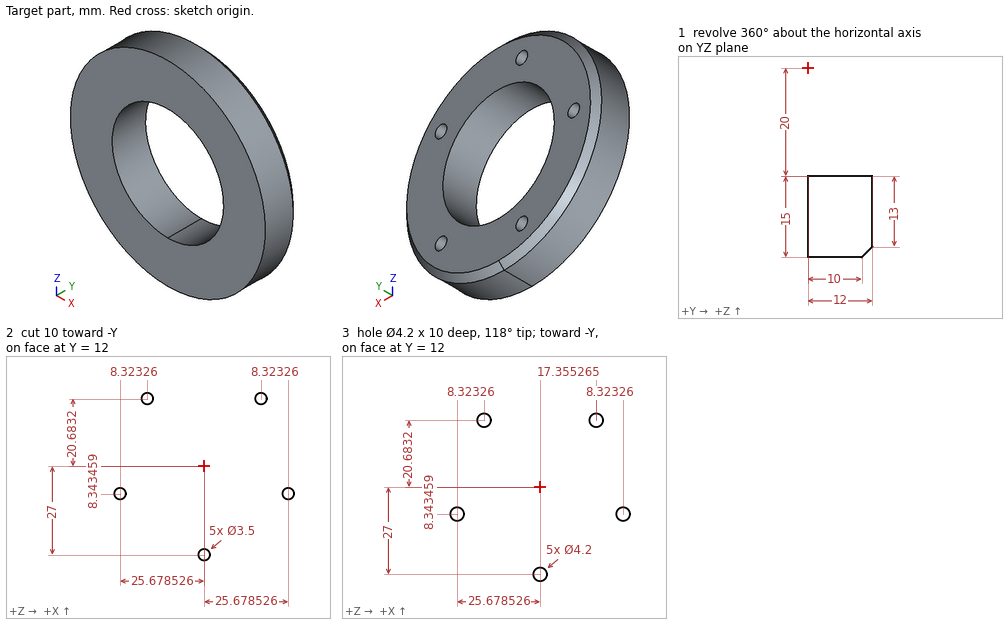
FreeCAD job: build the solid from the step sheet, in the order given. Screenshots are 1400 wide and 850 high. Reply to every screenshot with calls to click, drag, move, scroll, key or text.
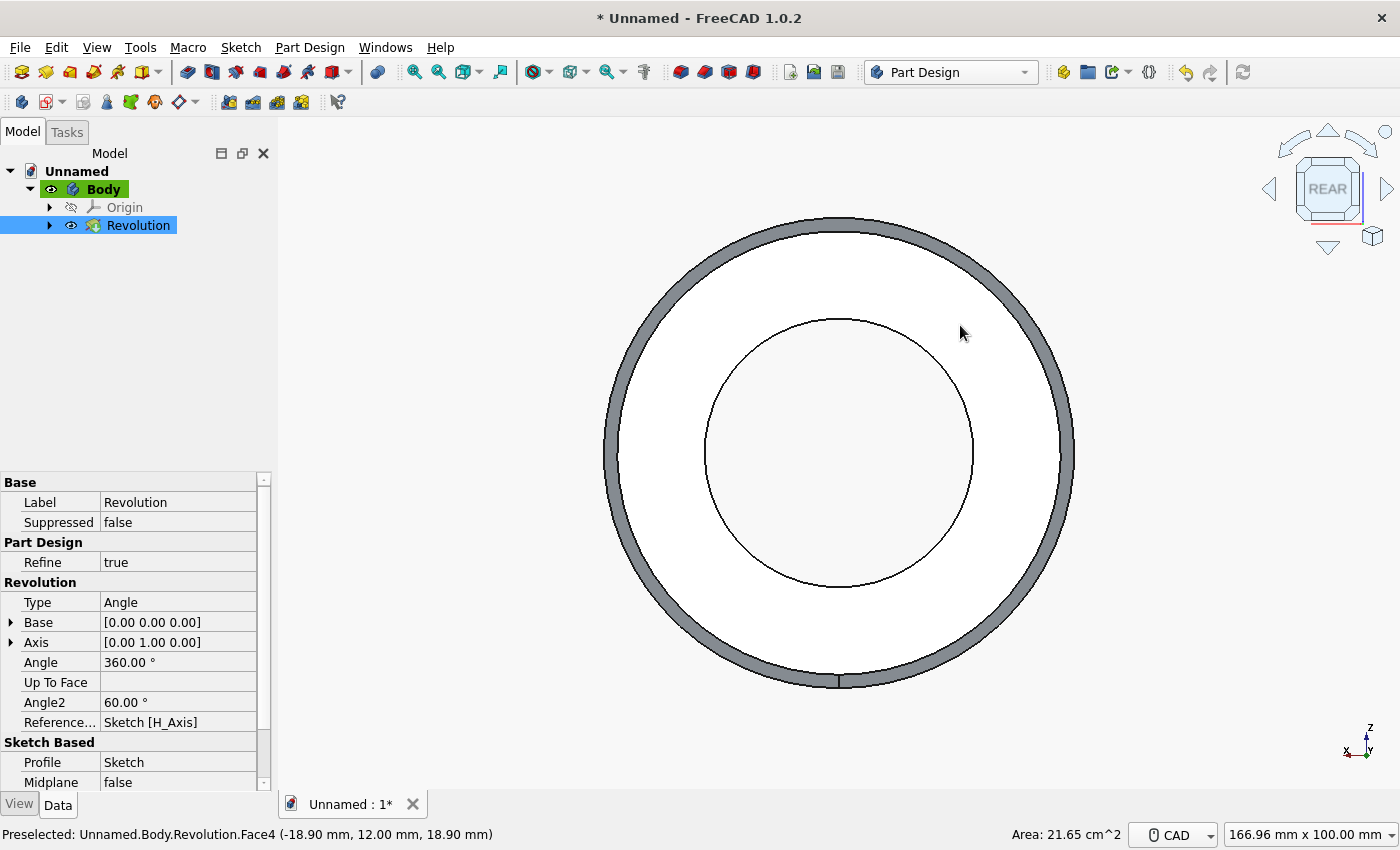
click(46, 102)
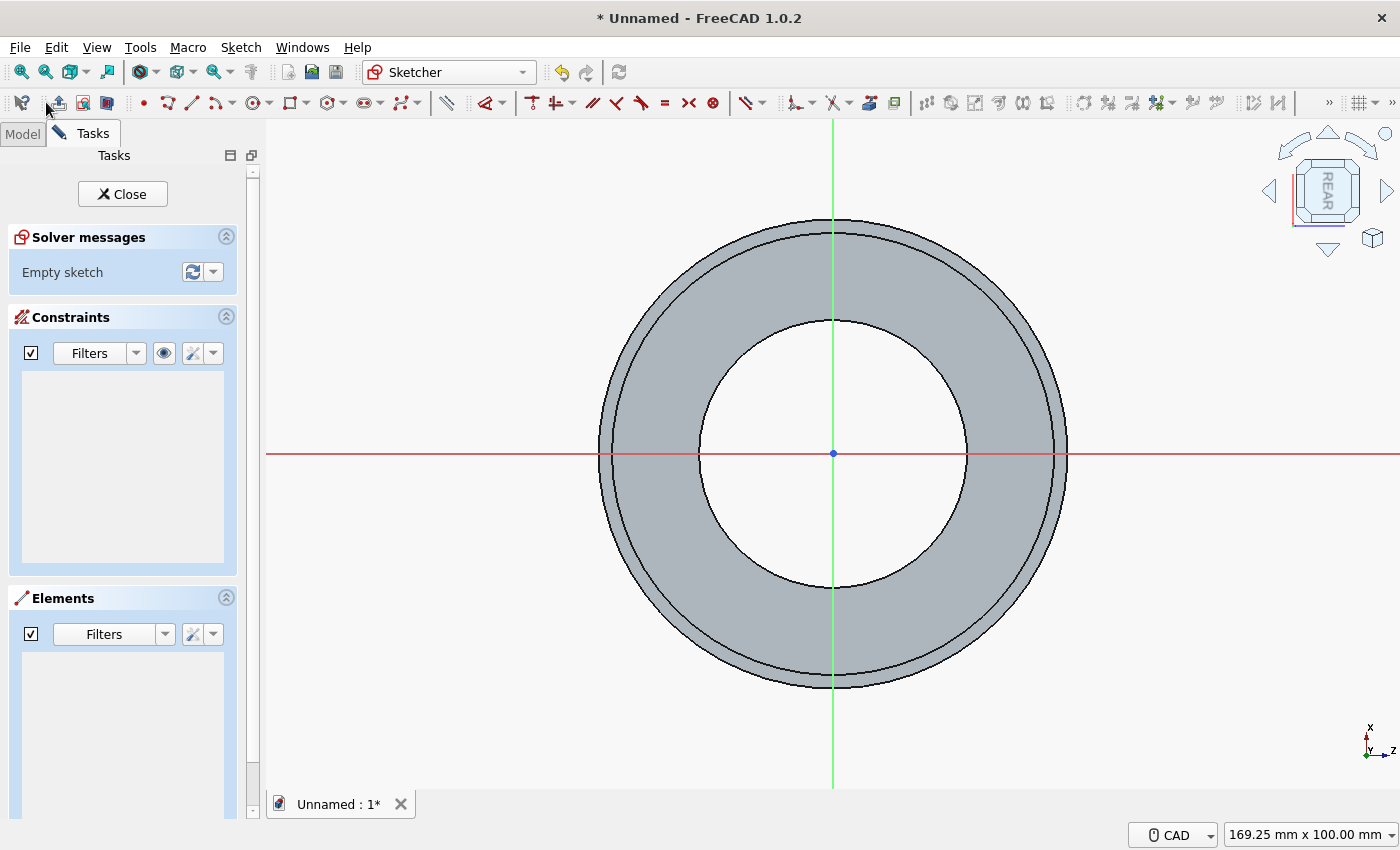
click(254, 104)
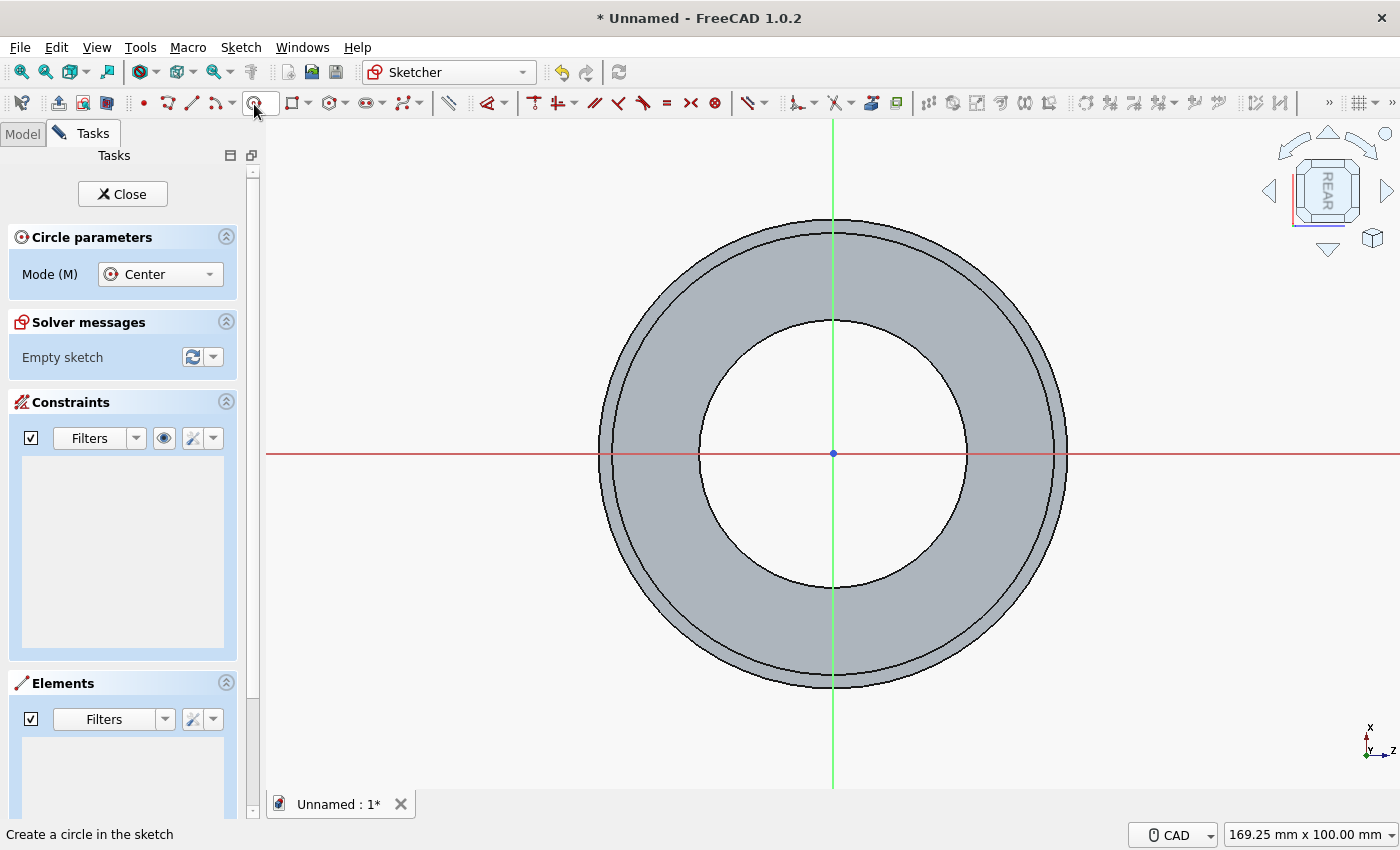
scroll(833, 635, up, 4)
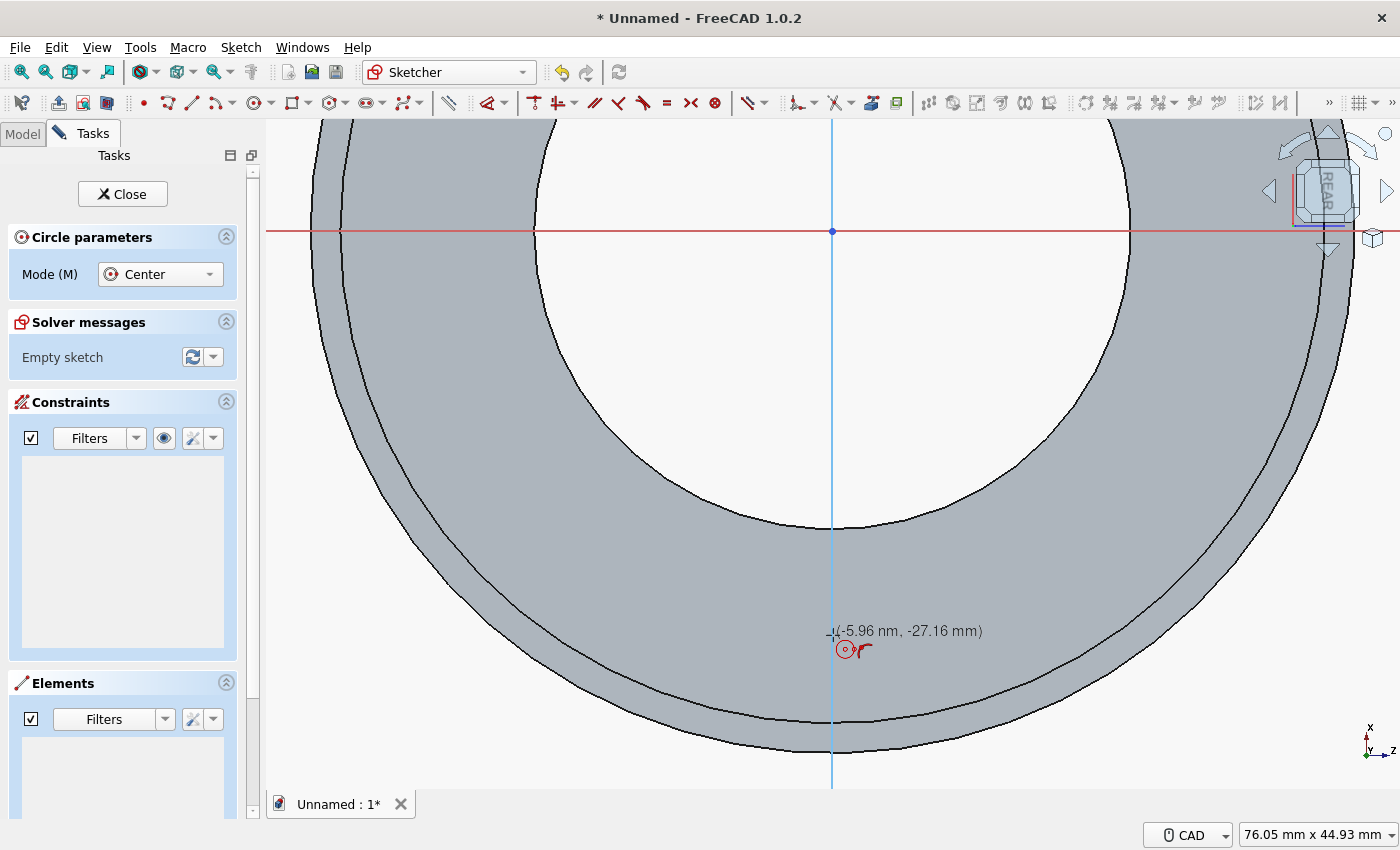
click(832, 634)
click(851, 615)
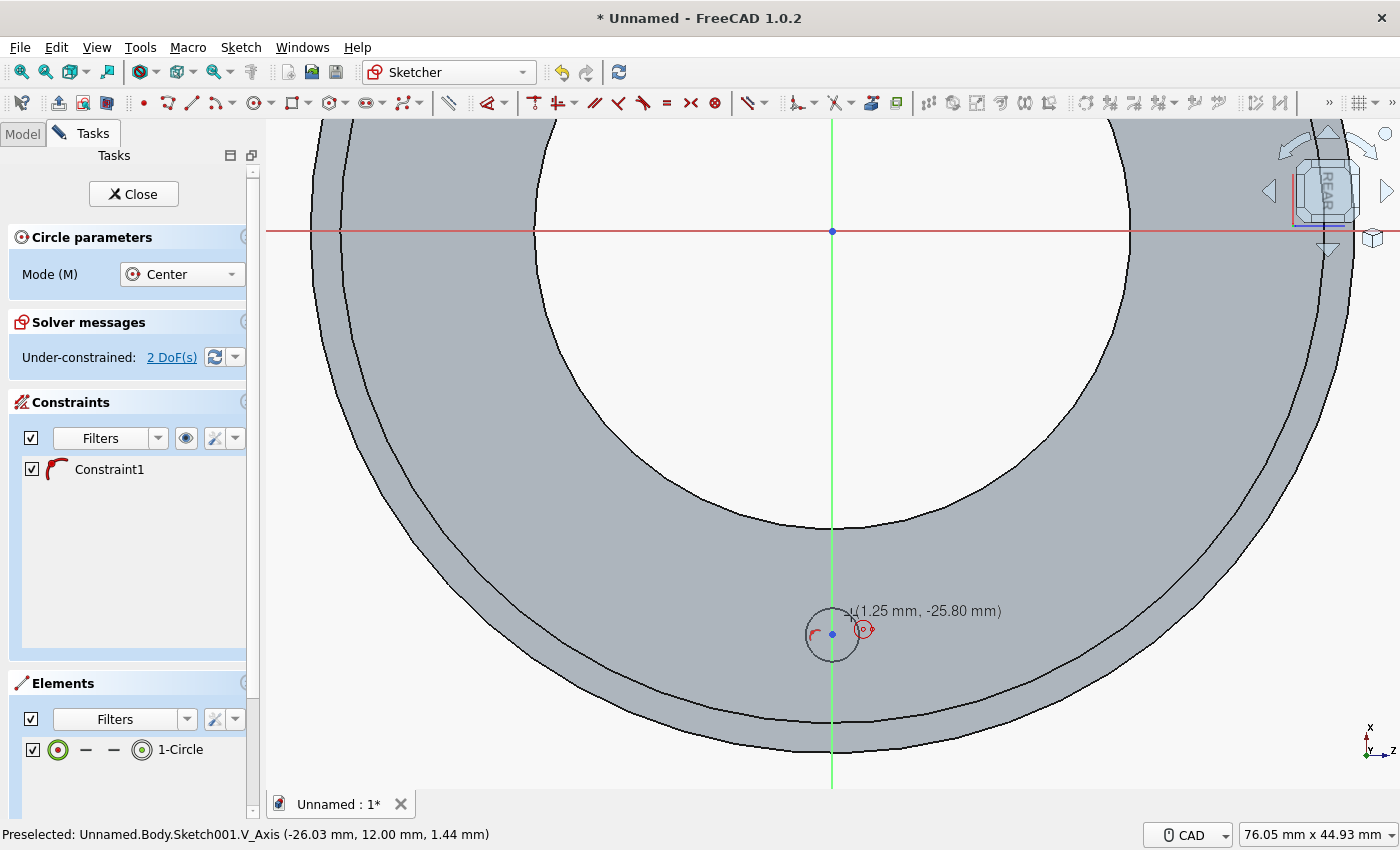
click(449, 356)
click(468, 337)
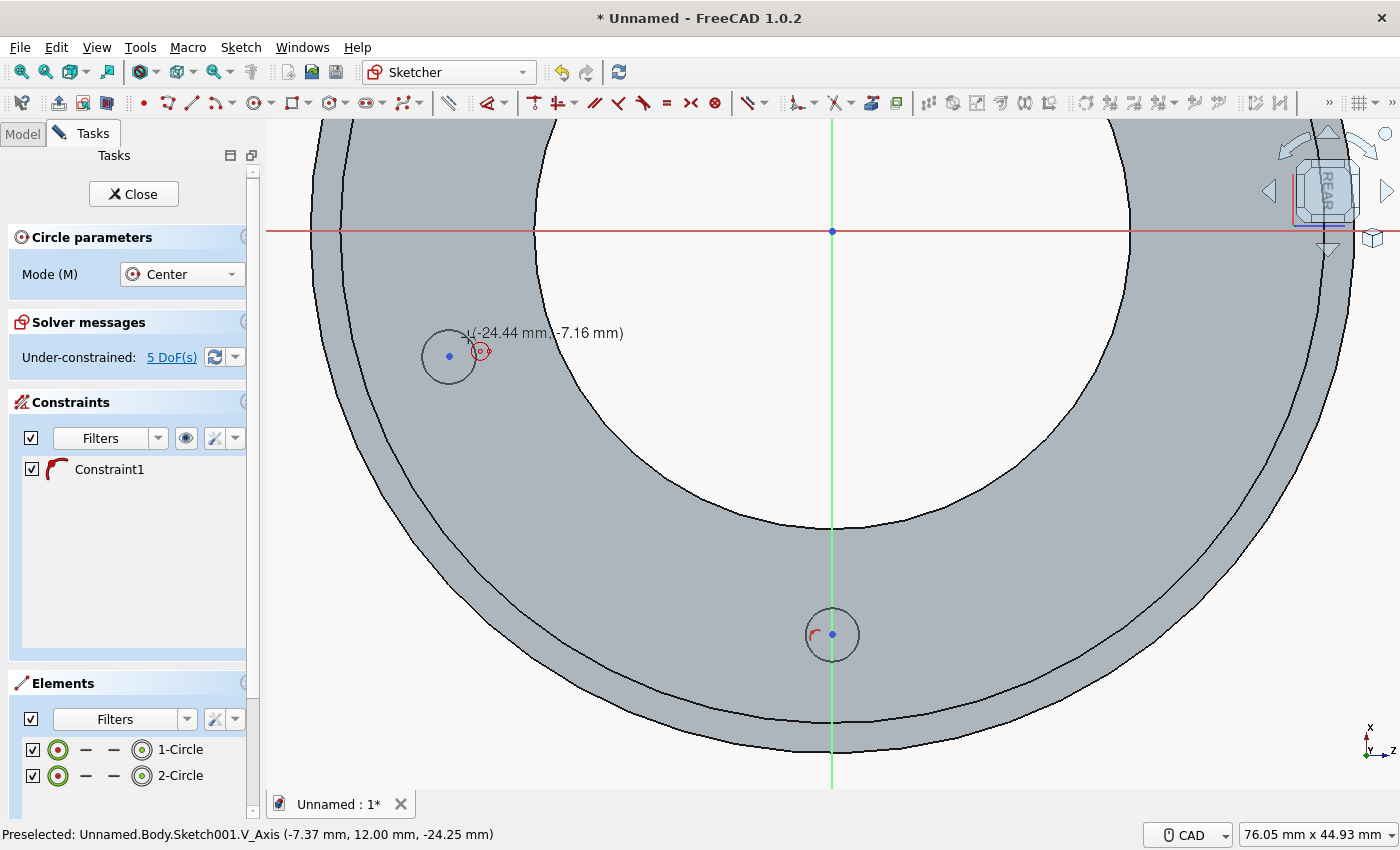
click(1215, 356)
click(1234, 337)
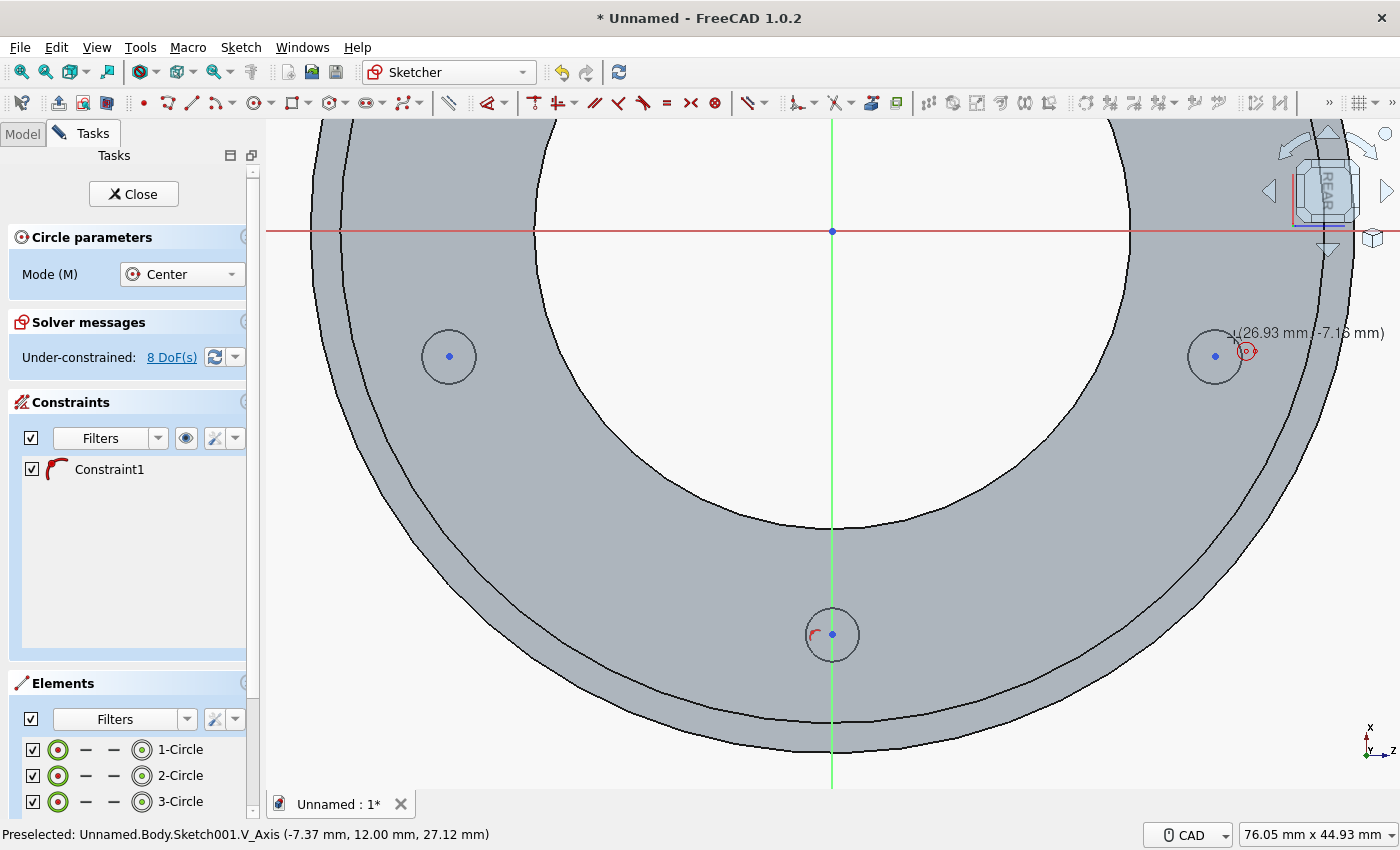
scroll(682, 668, down, 3)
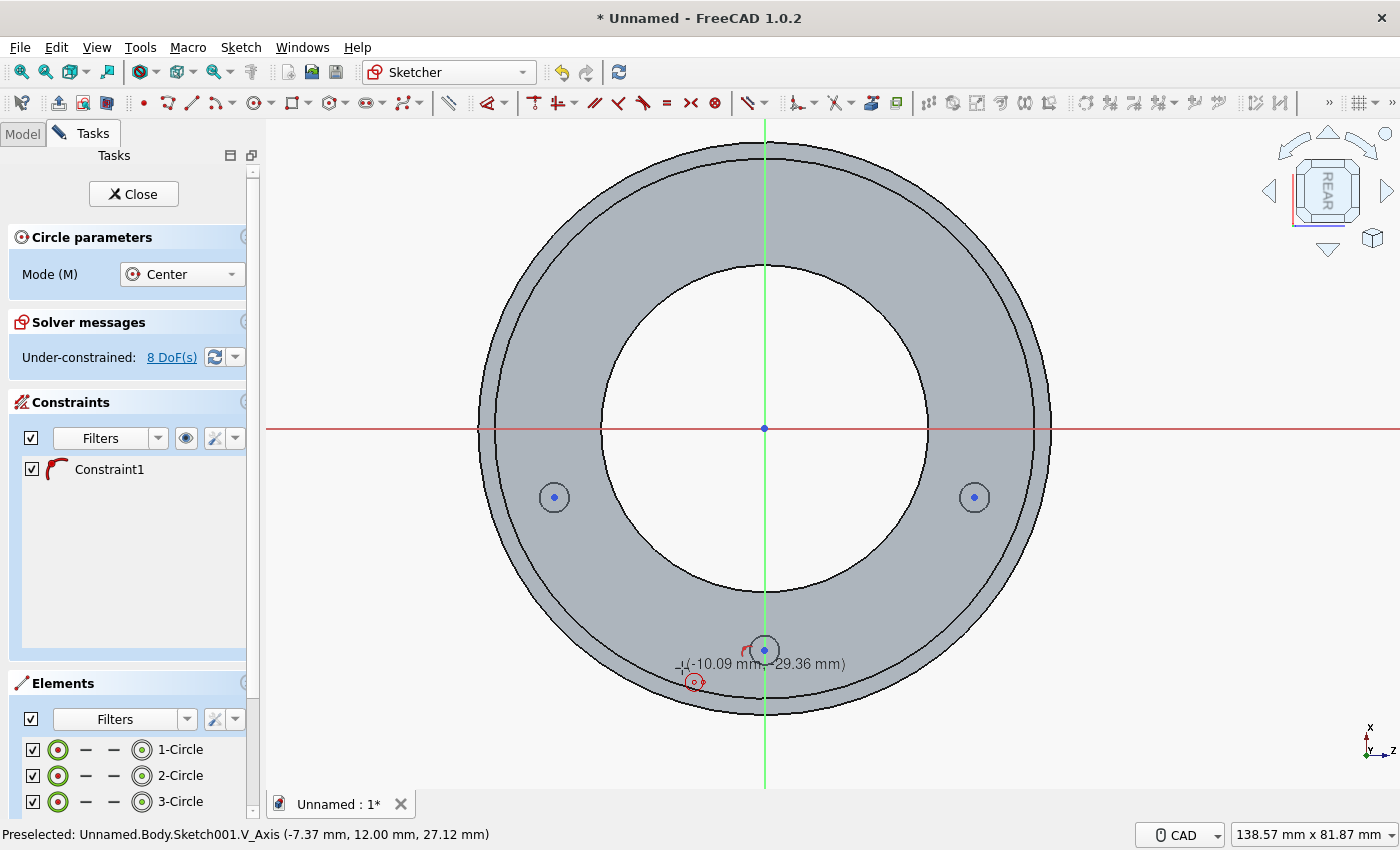
scroll(623, 259, up, 3)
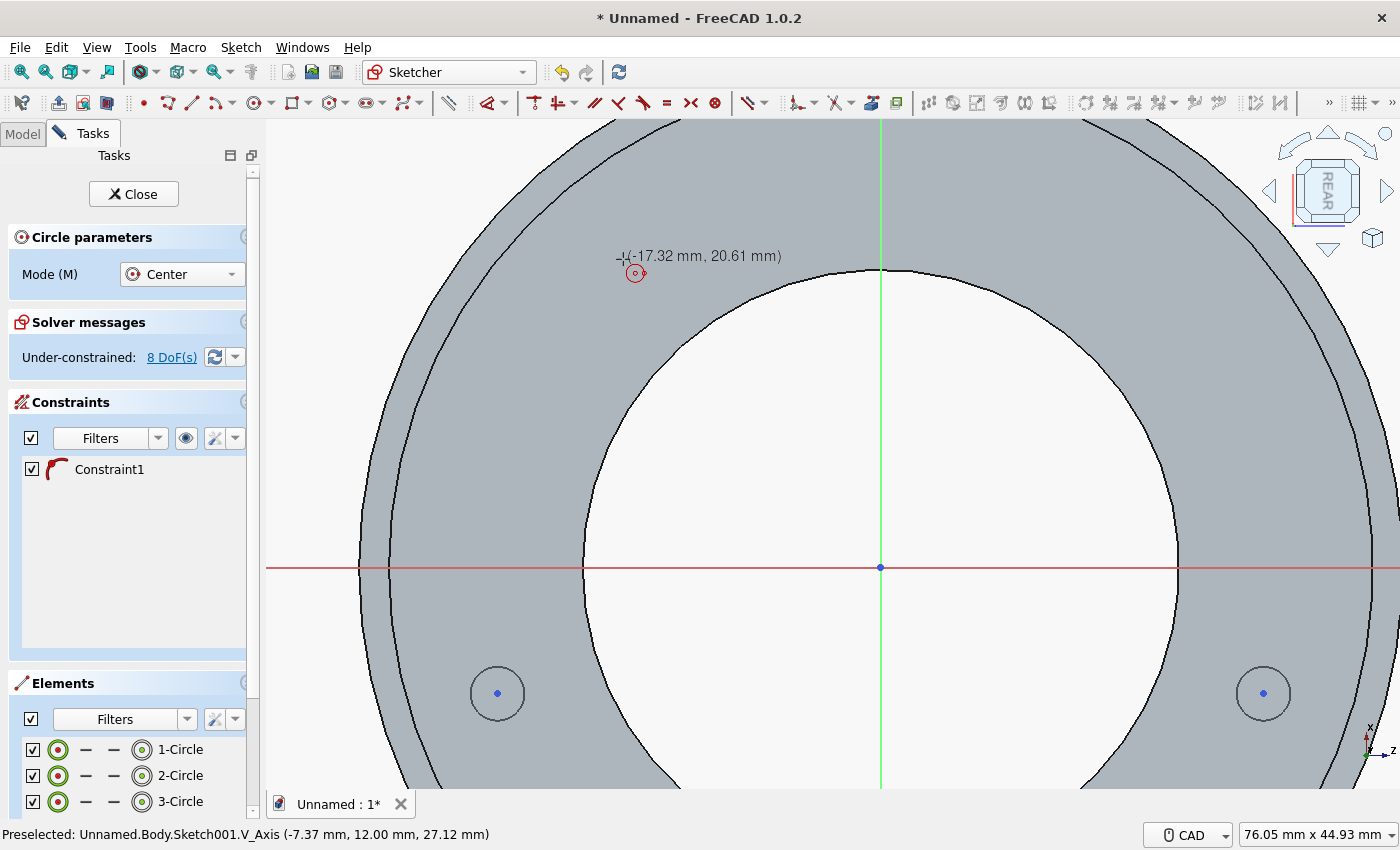
click(622, 260)
click(641, 241)